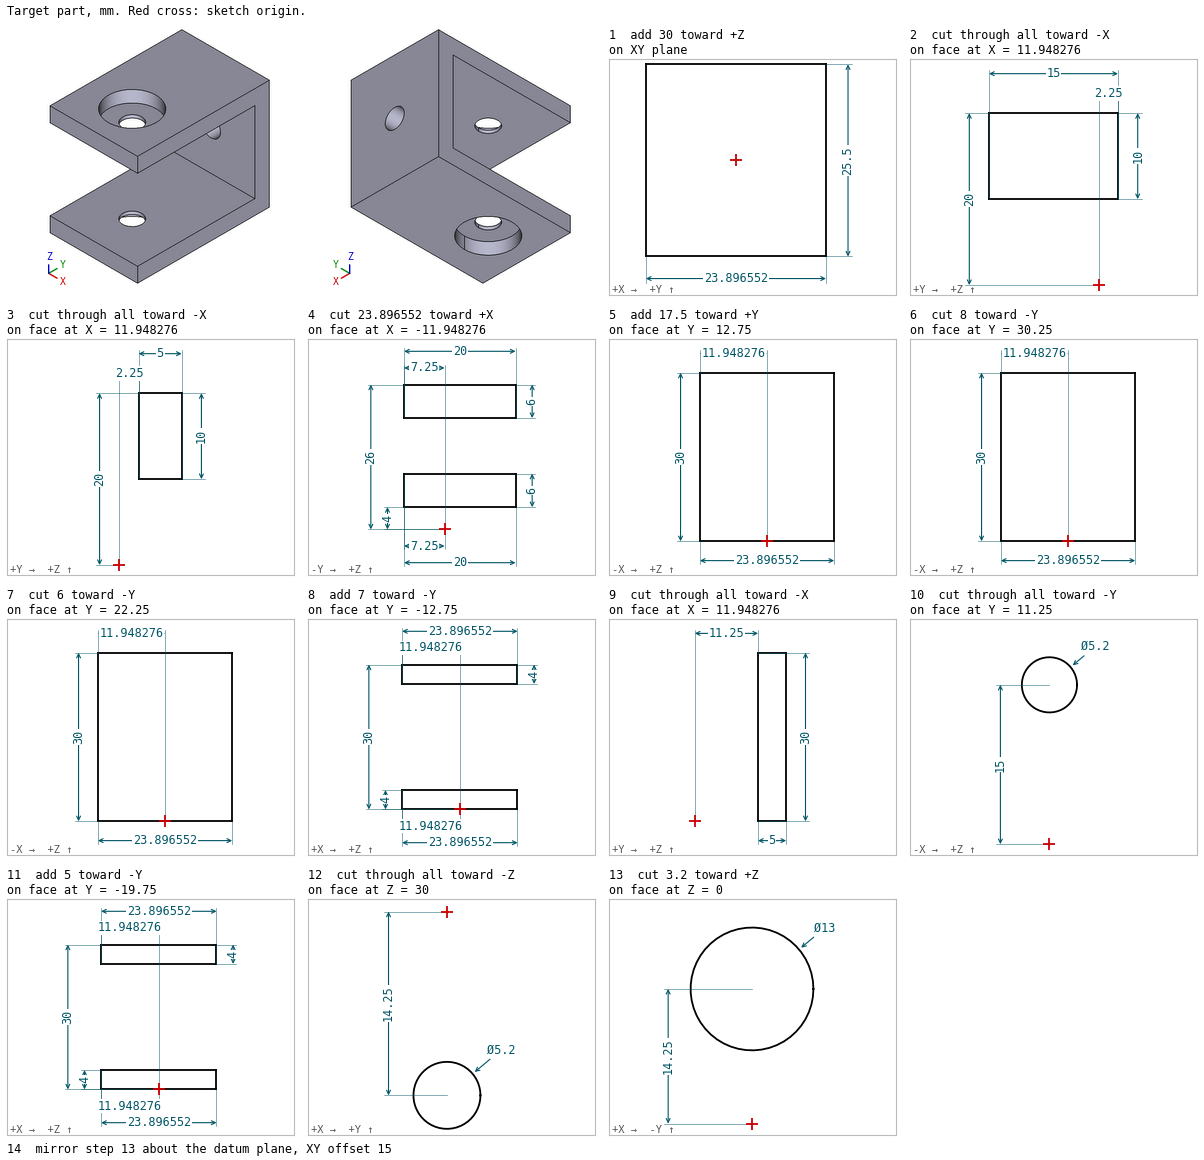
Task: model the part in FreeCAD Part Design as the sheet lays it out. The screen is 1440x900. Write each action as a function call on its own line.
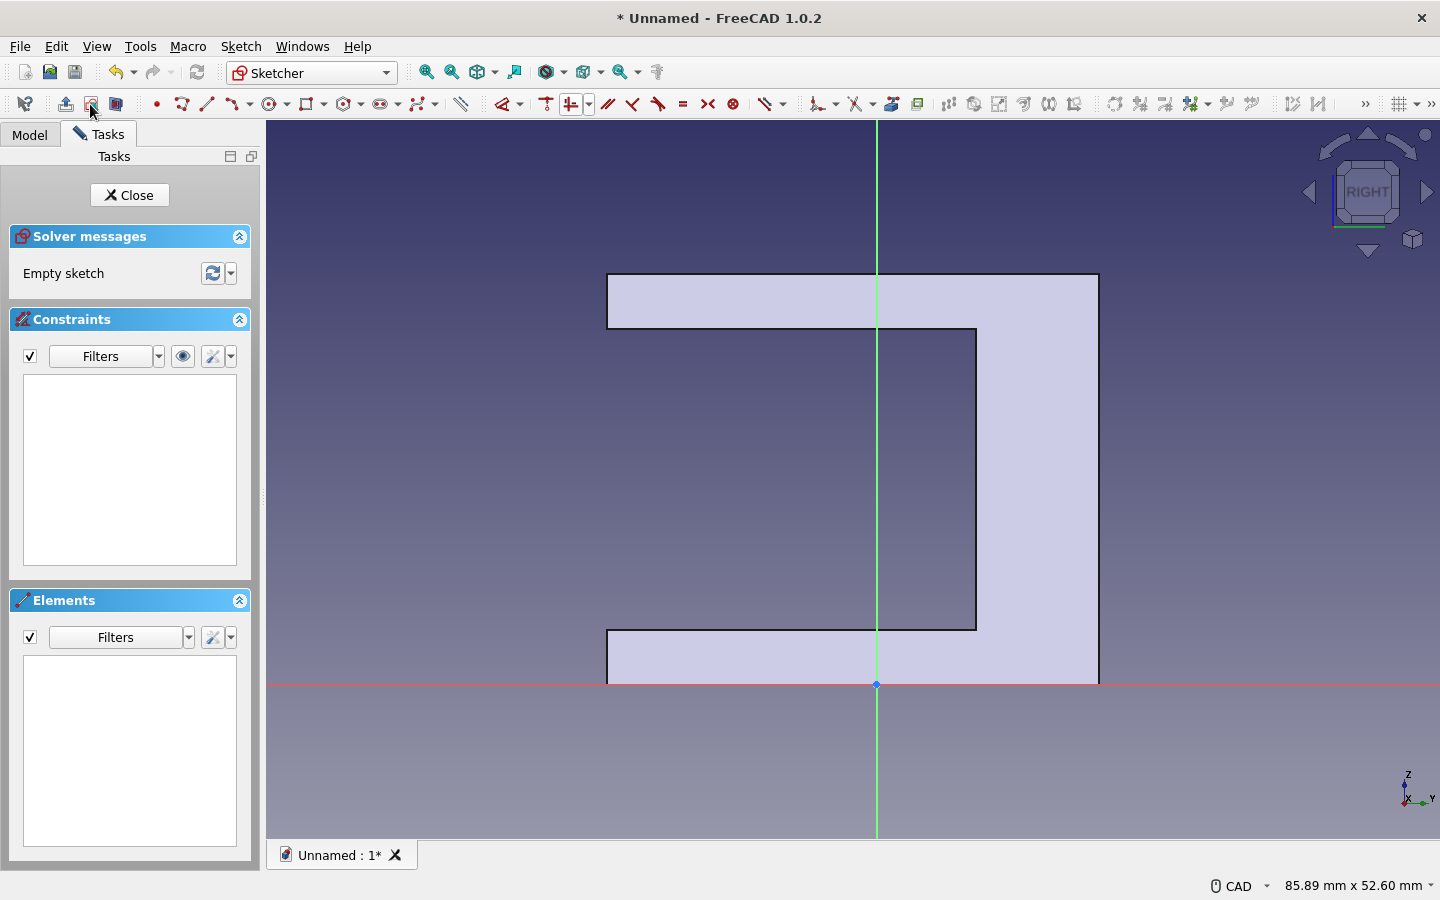
key(g)
key(r)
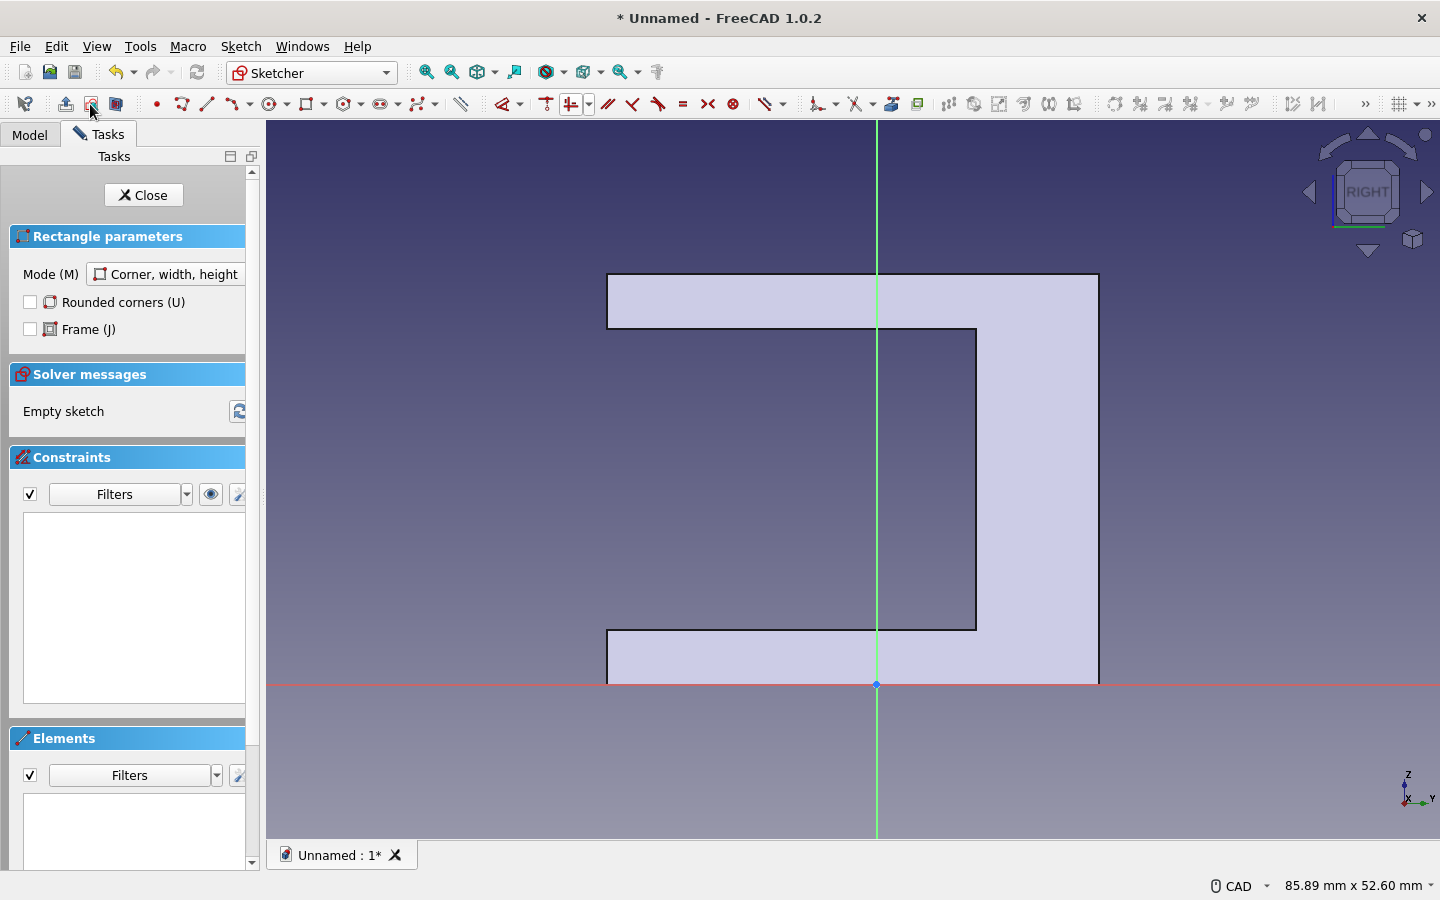
click(1031, 274)
click(1099, 685)
key(Escape)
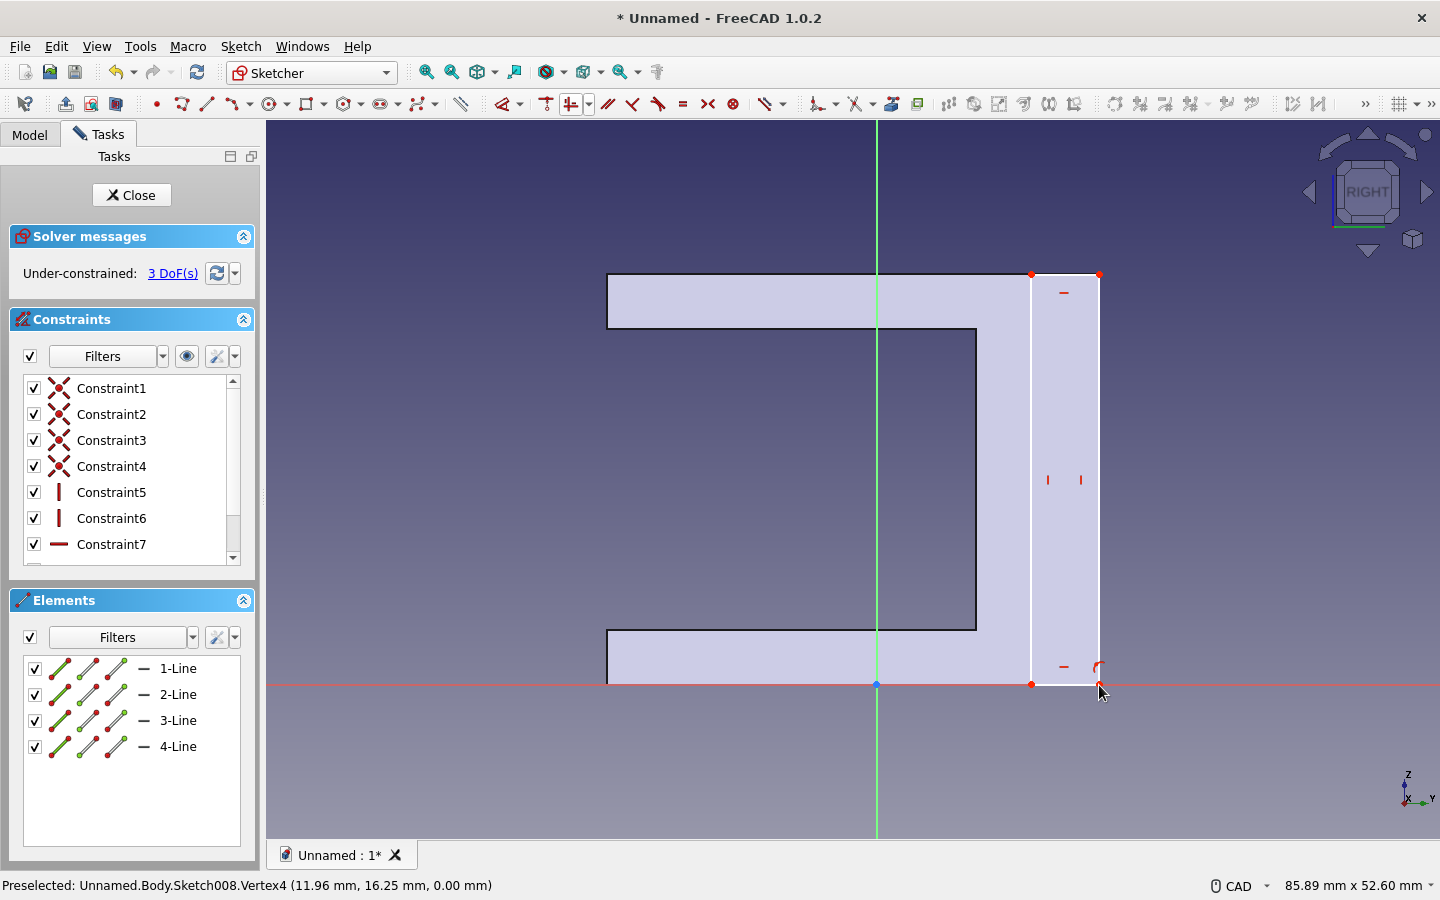
key(d)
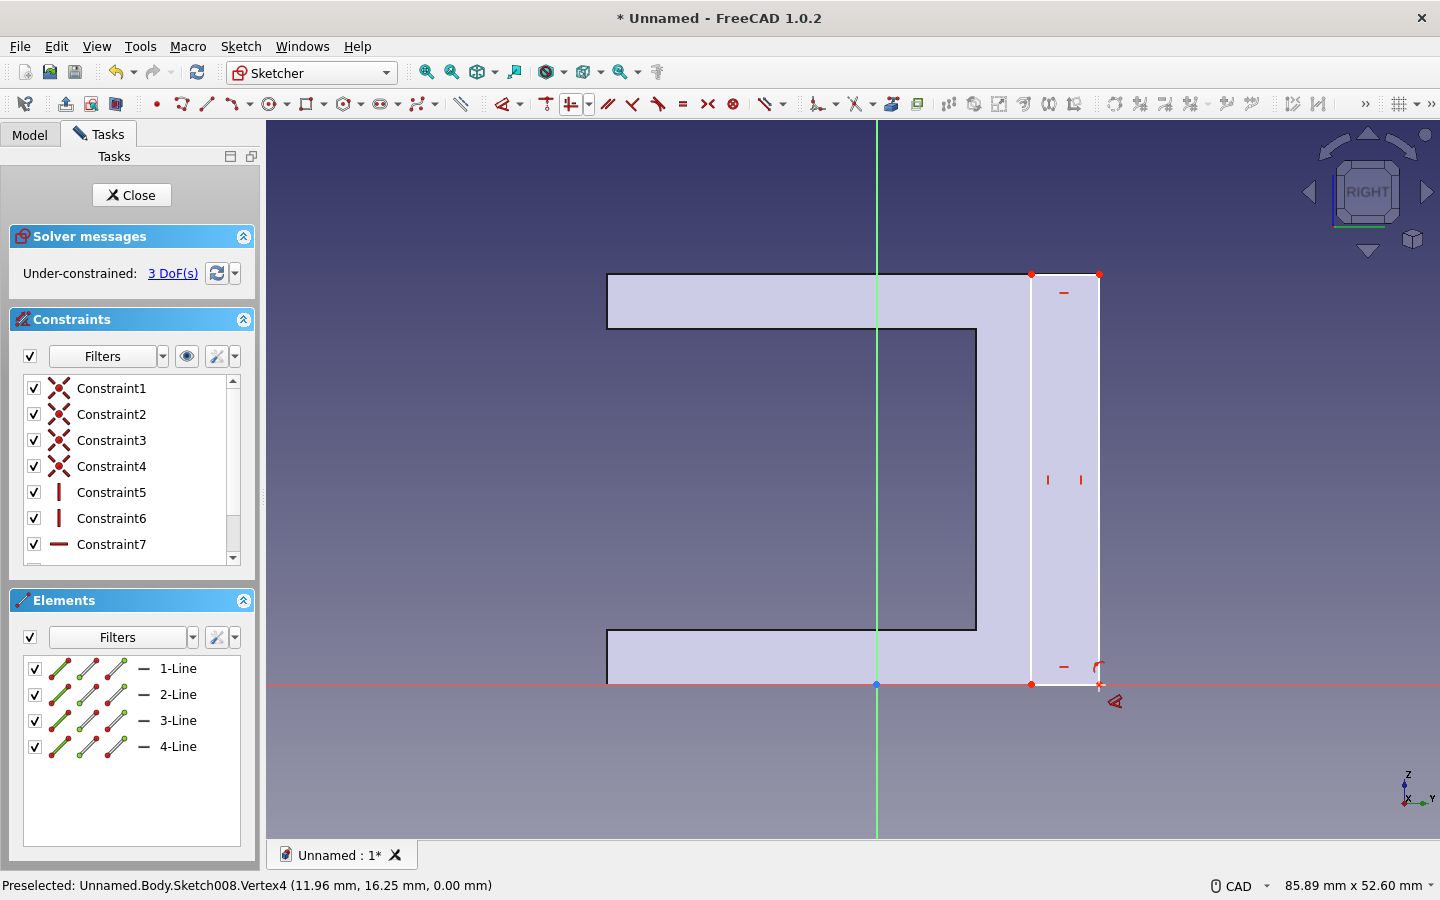
click(1051, 685)
click(1065, 719)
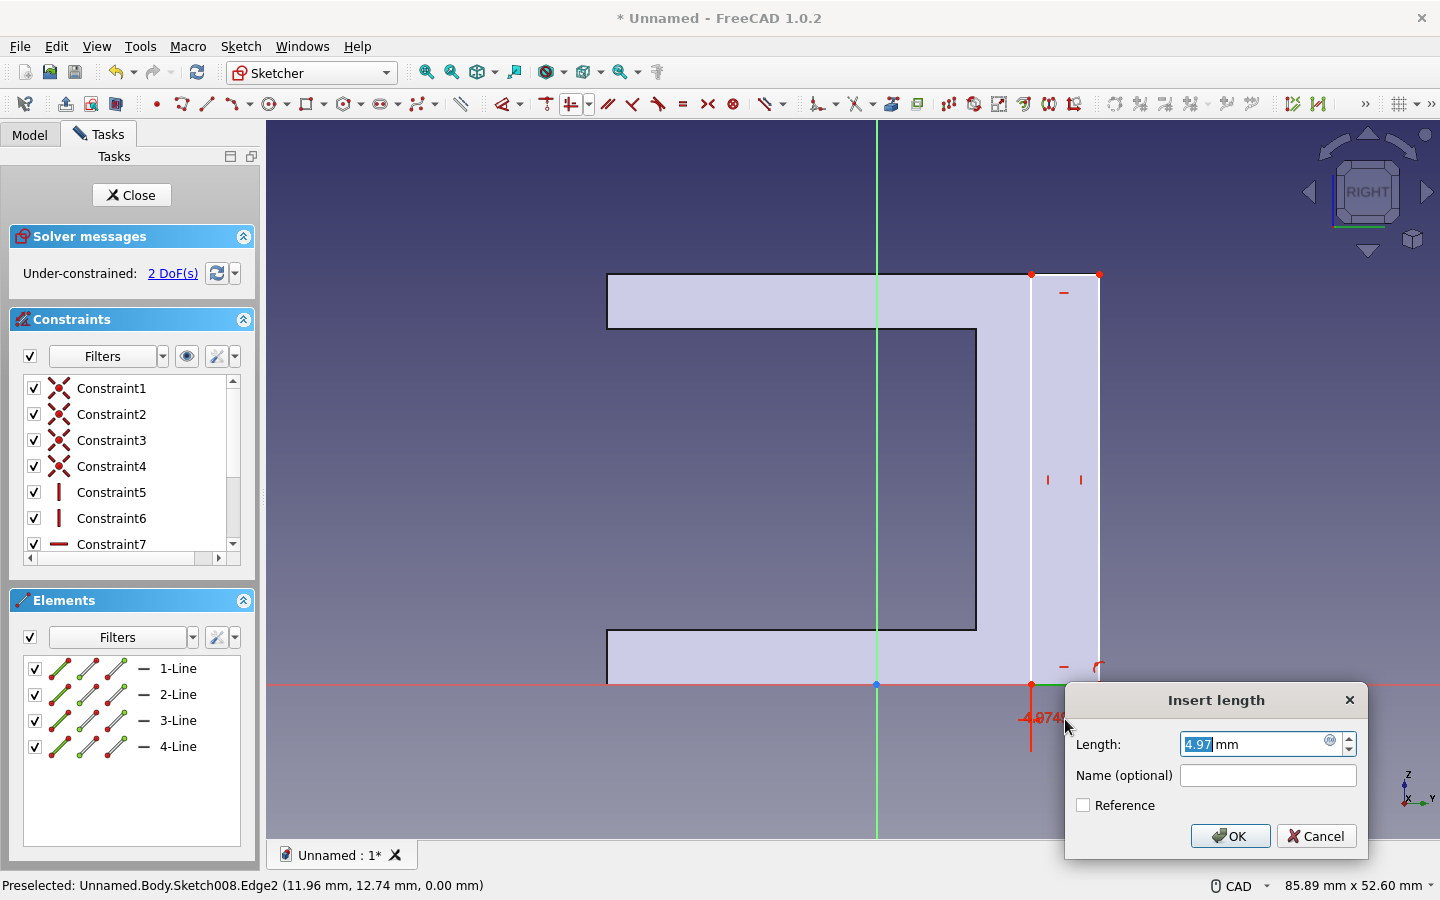
text(5)
key(Return)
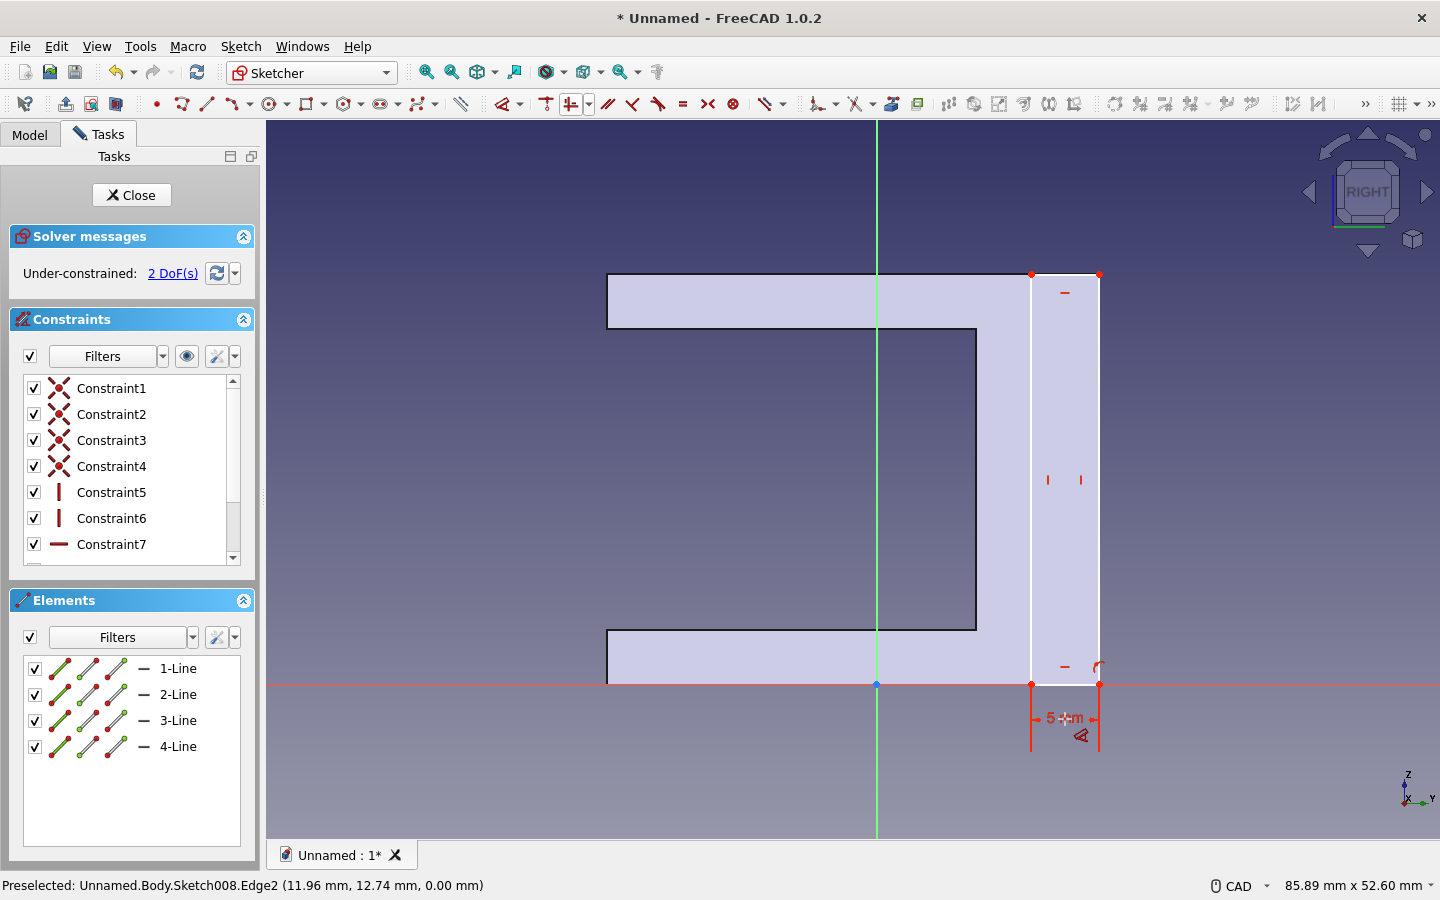
click(1031, 398)
click(1065, 480)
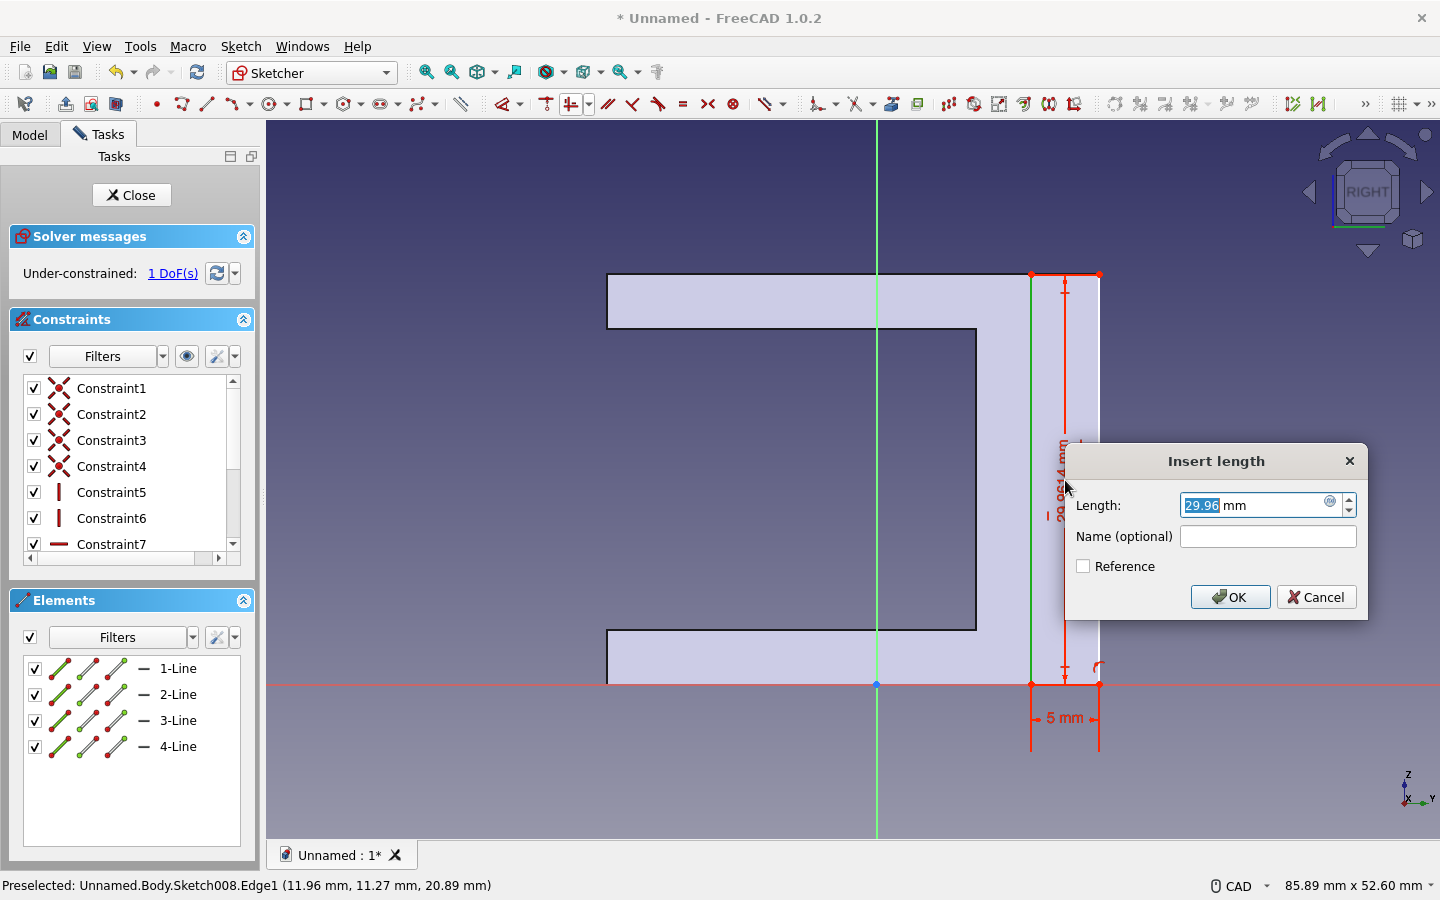
text(30)
key(Return)